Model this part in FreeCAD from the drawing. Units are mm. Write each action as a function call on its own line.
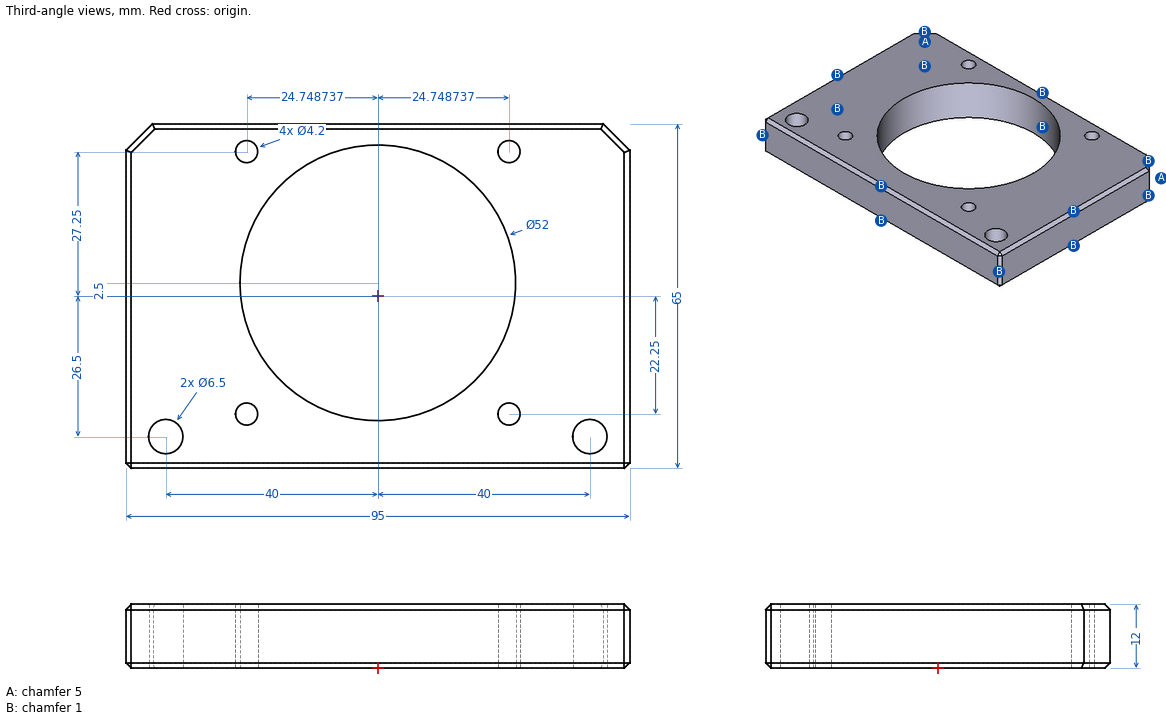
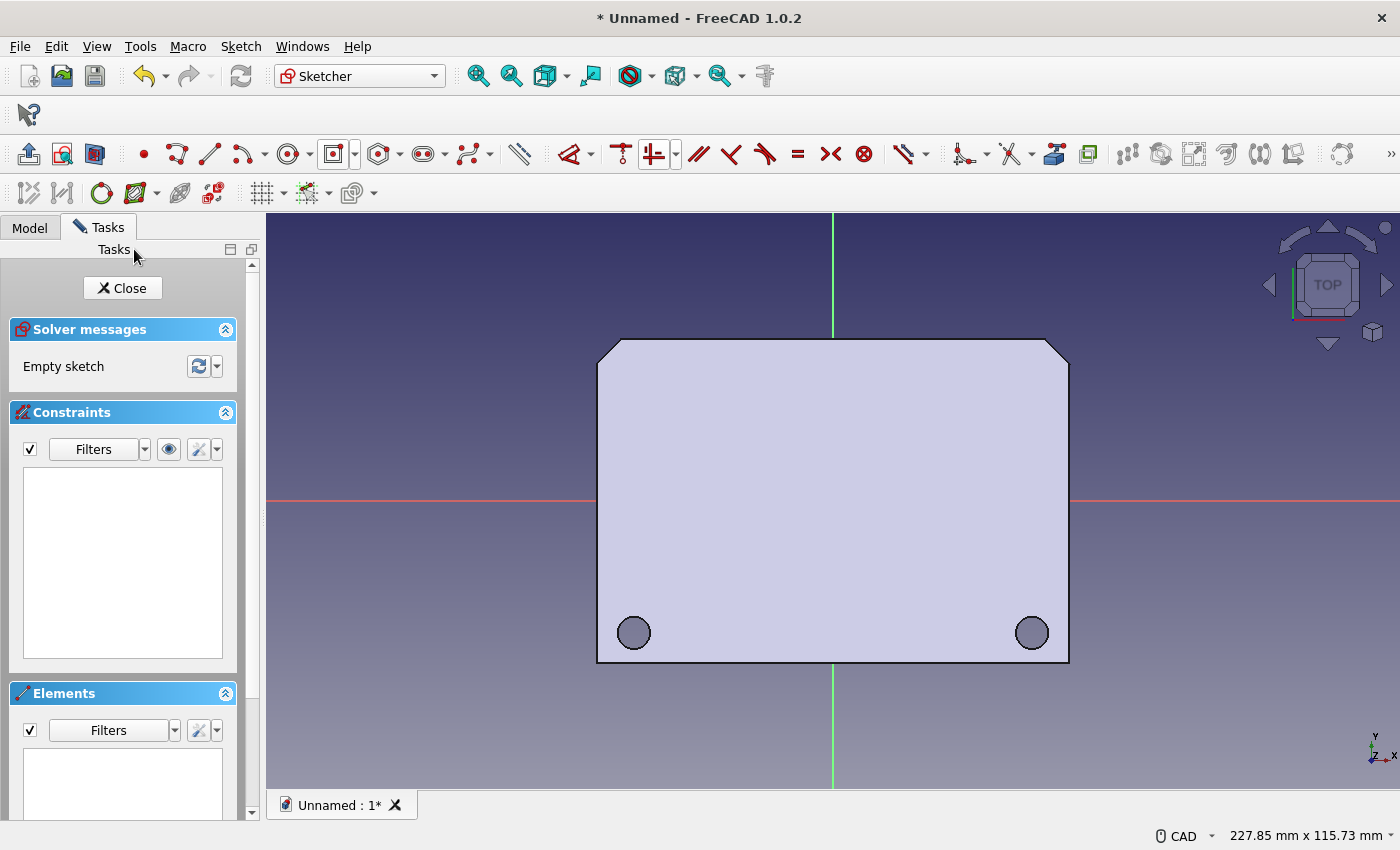
click(95, 154)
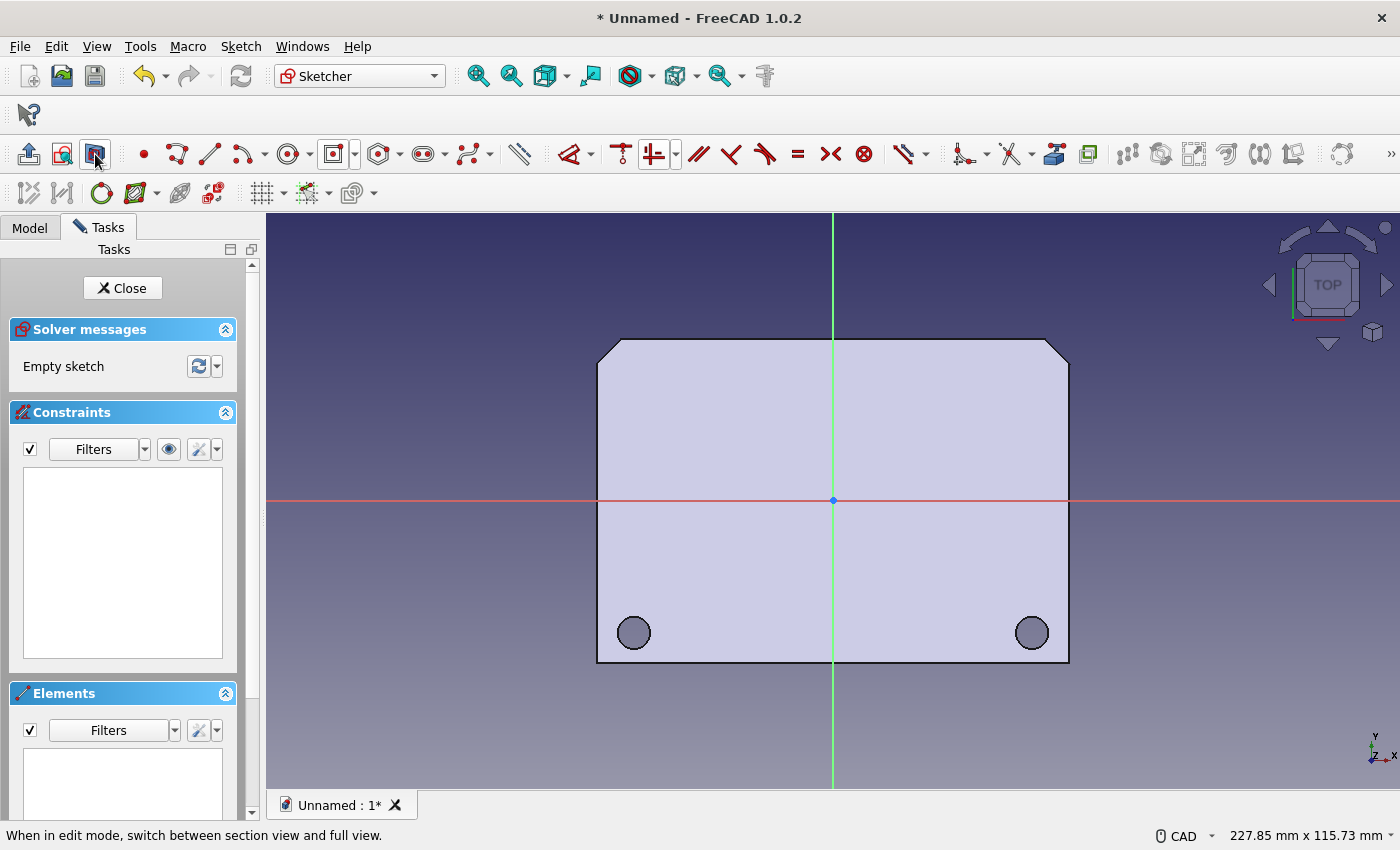
scroll(972, 463, up, 2)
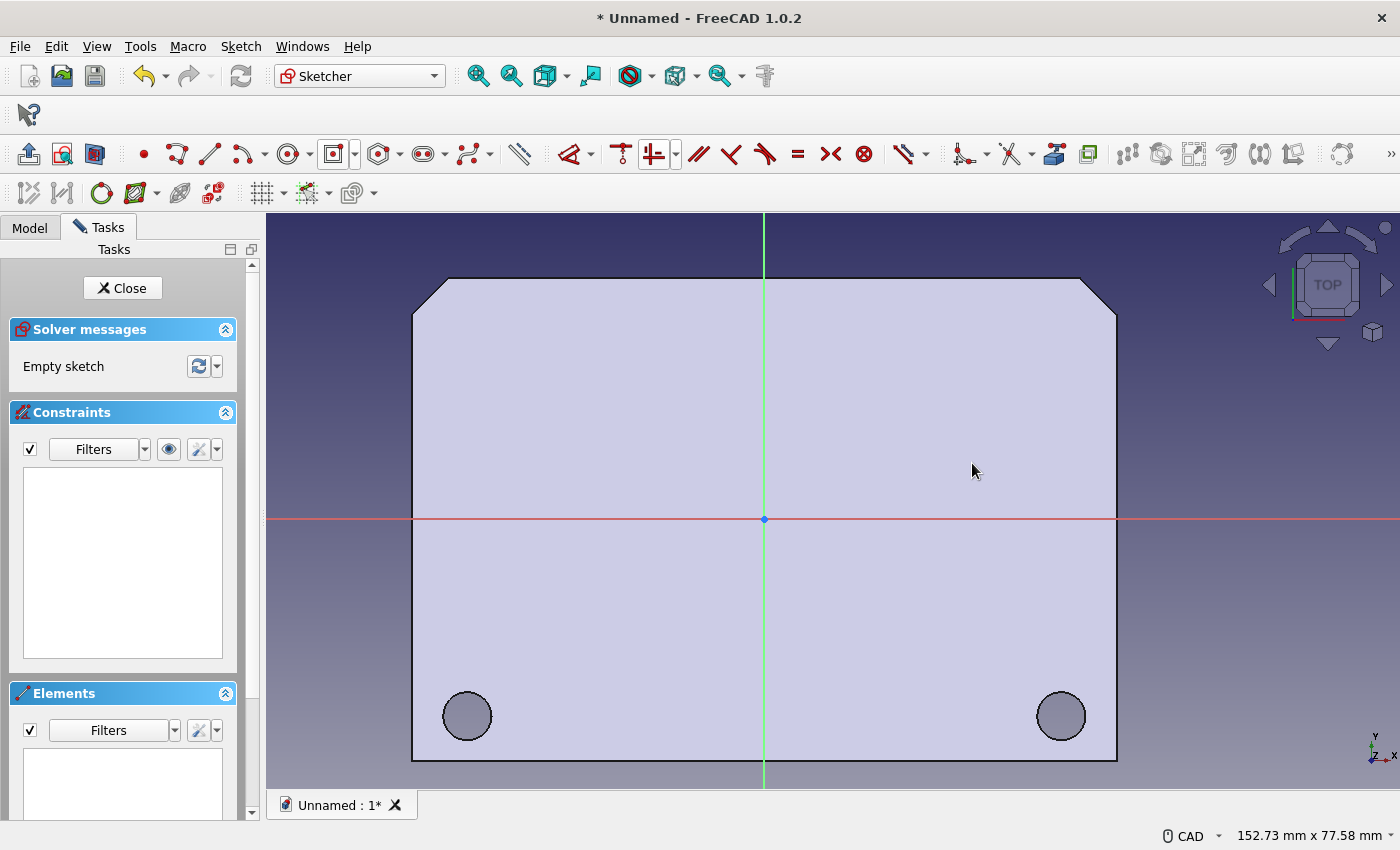
click(288, 154)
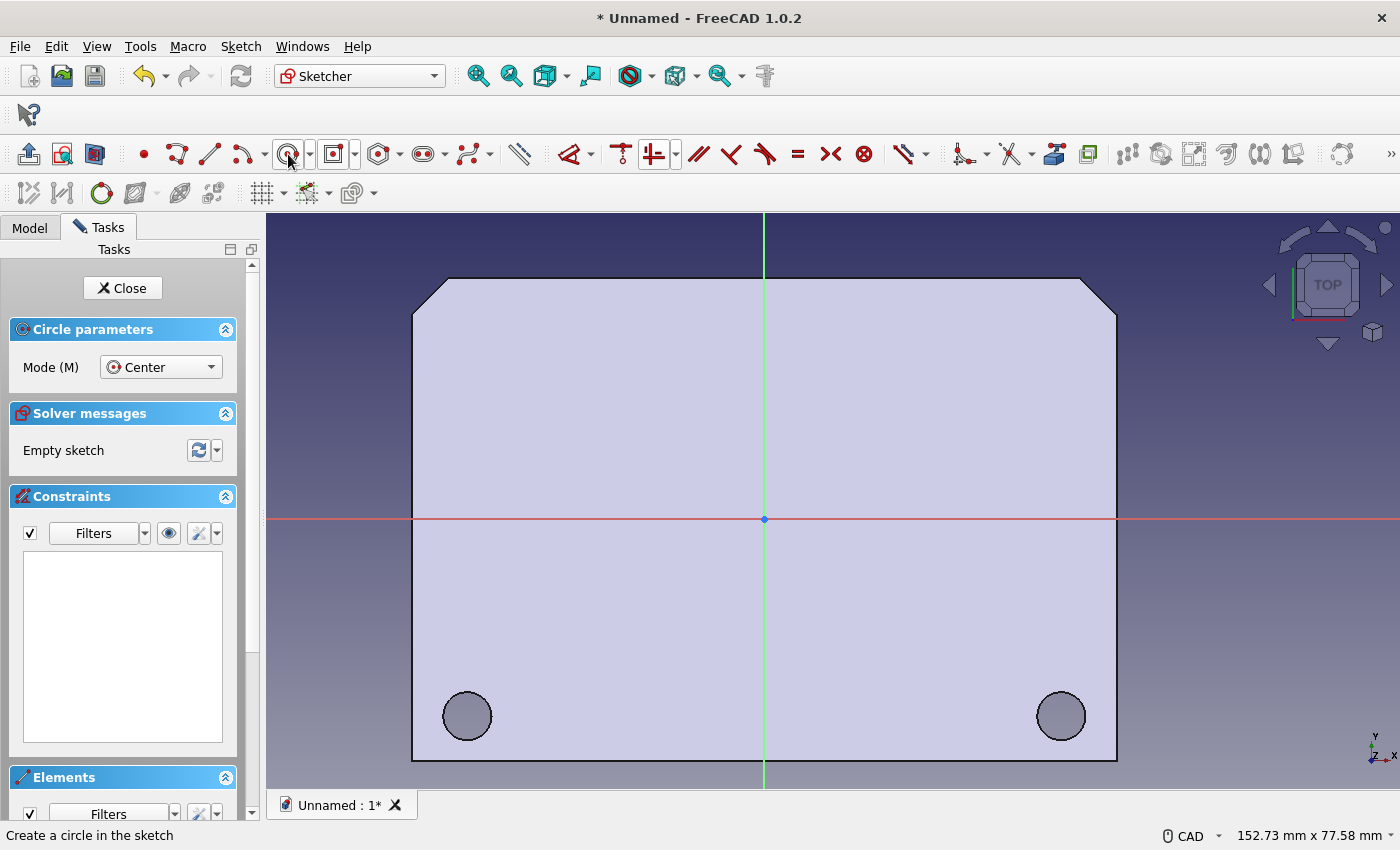
click(764, 501)
click(901, 364)
key(Escape)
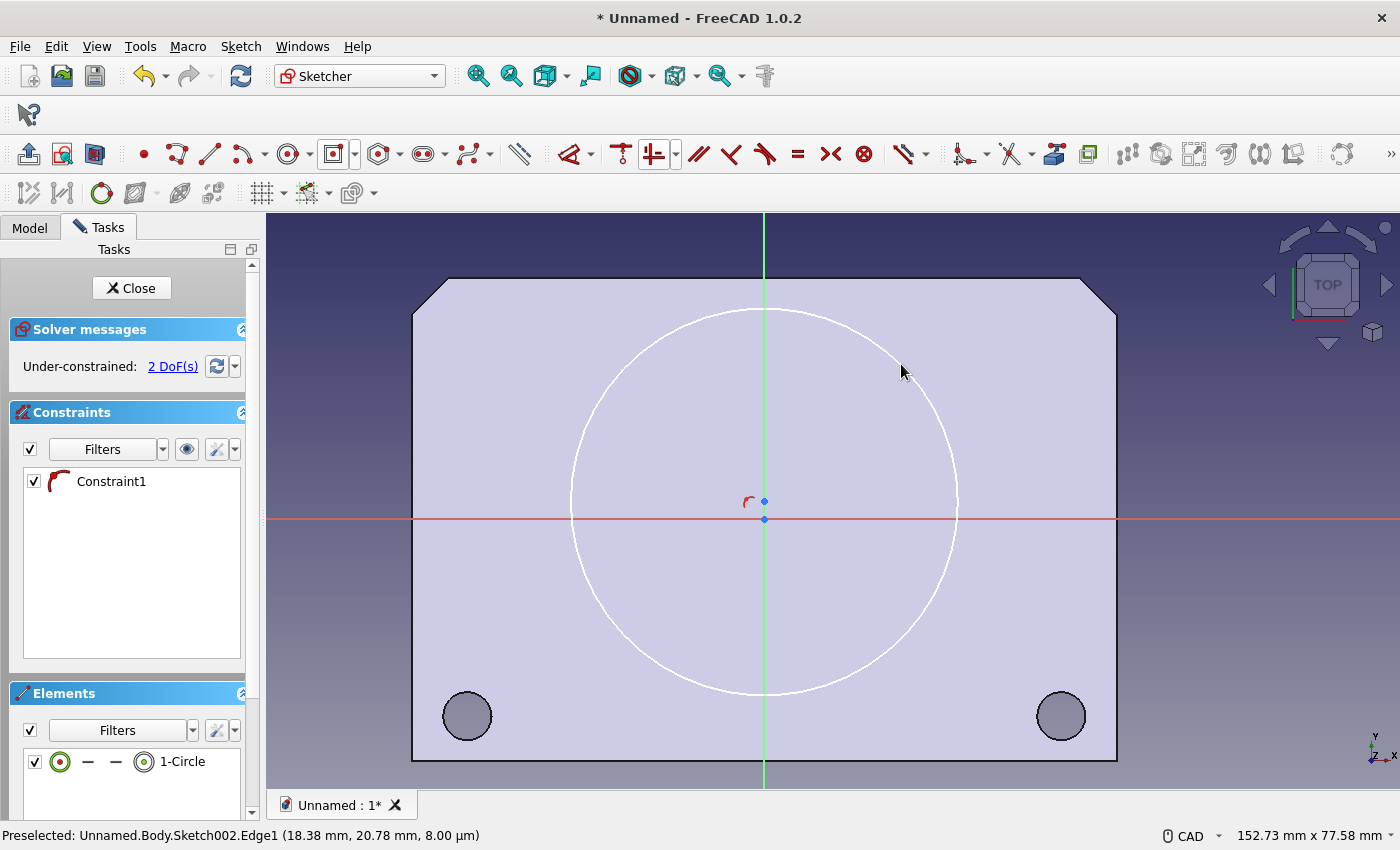
click(568, 154)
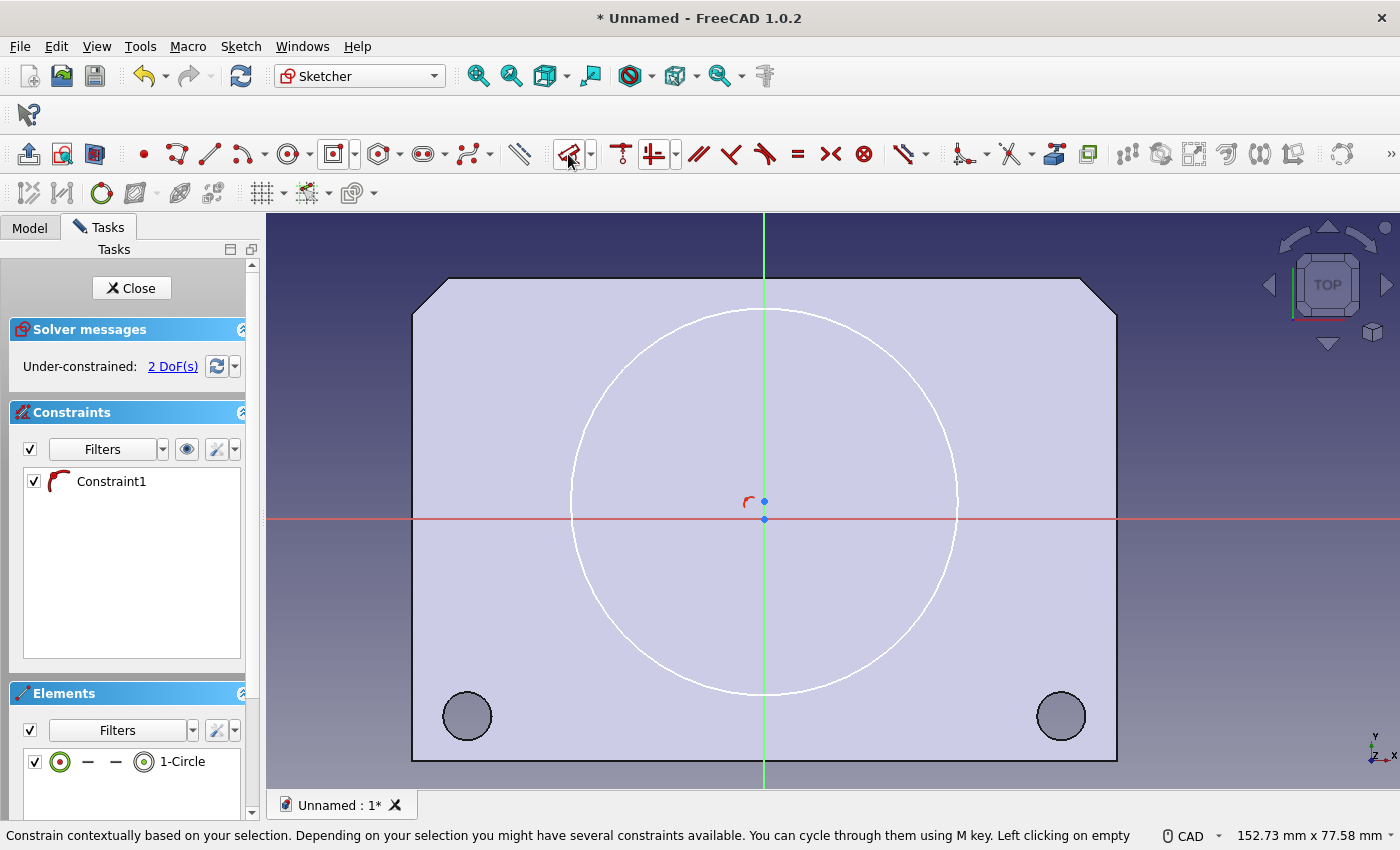
click(901, 365)
click(924, 342)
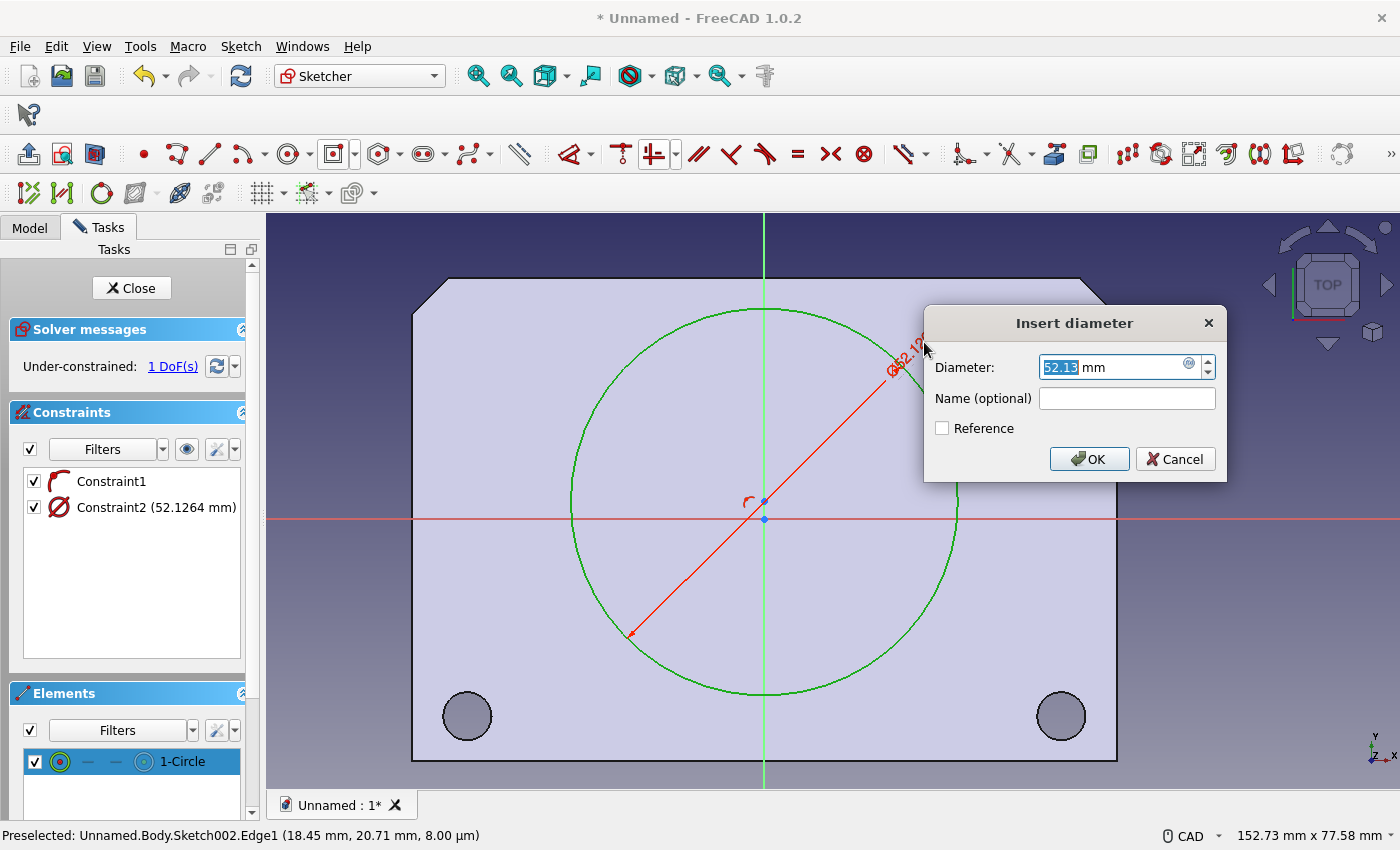
text(52)
key(Return)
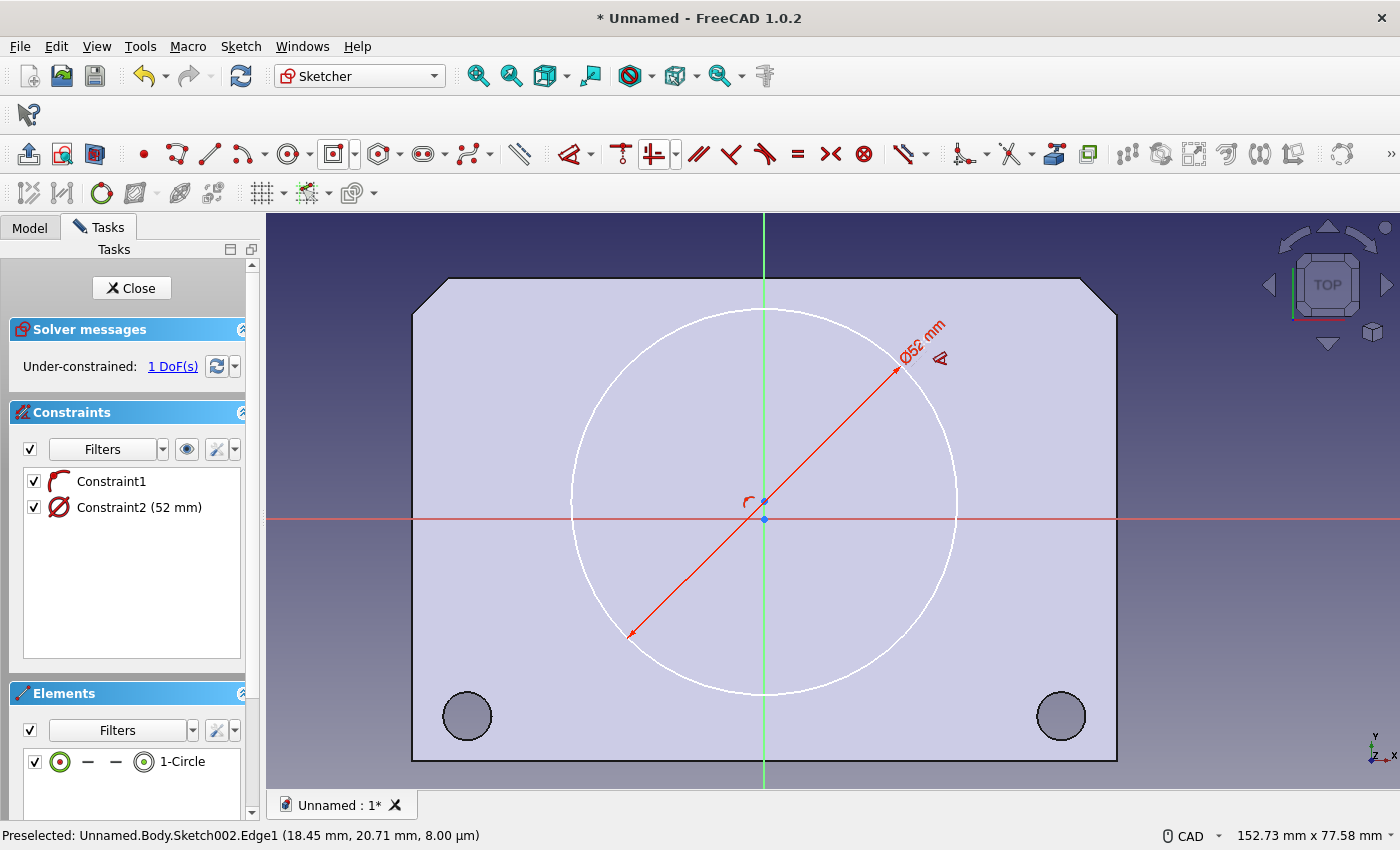
scroll(764, 502, up, 4)